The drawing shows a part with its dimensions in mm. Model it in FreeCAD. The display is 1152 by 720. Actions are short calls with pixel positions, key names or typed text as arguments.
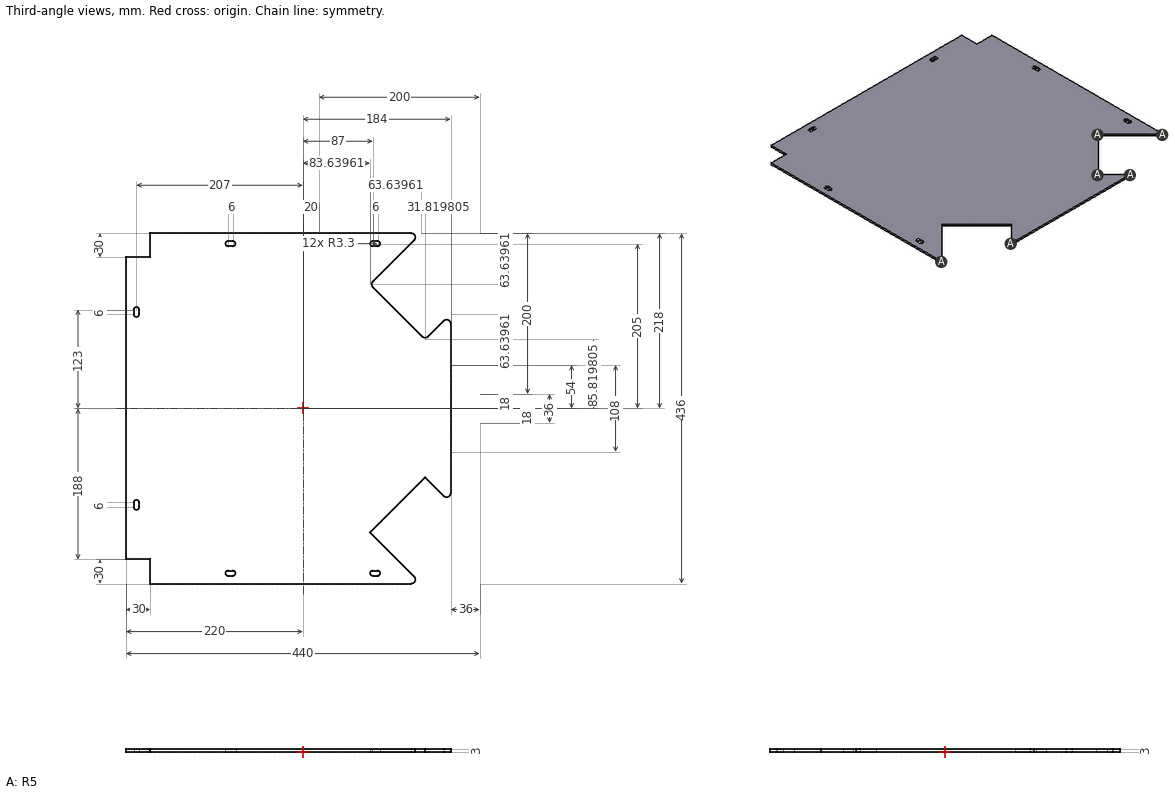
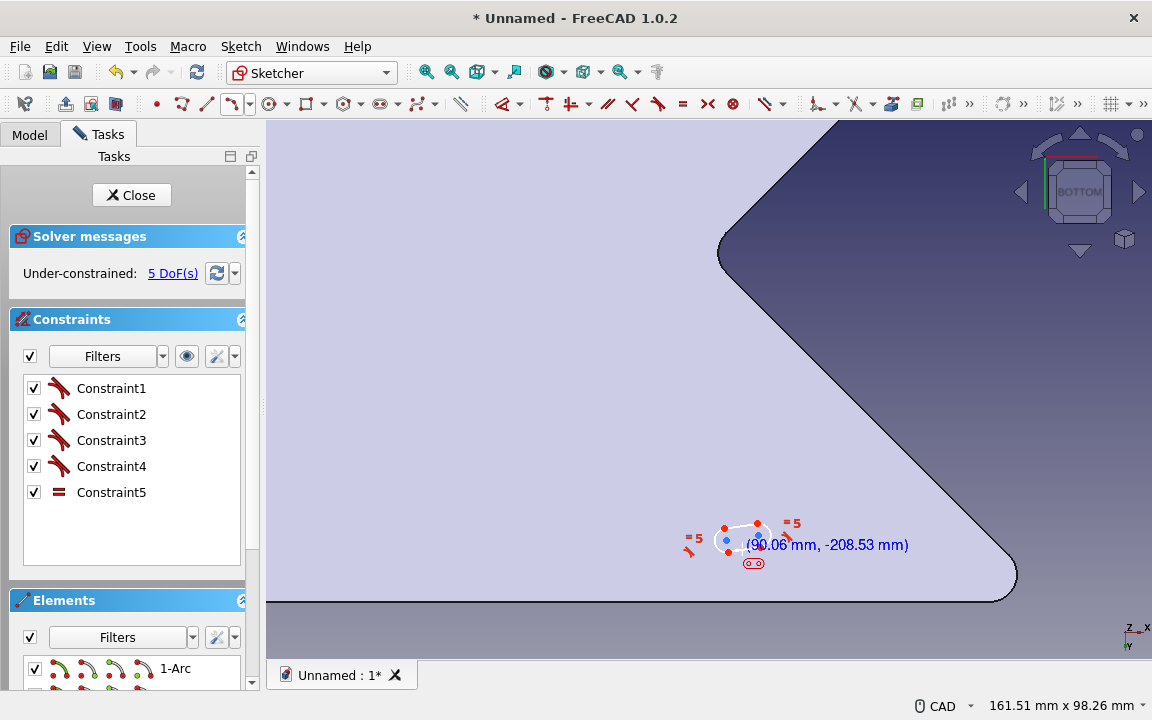
scroll(751, 543, down, 10)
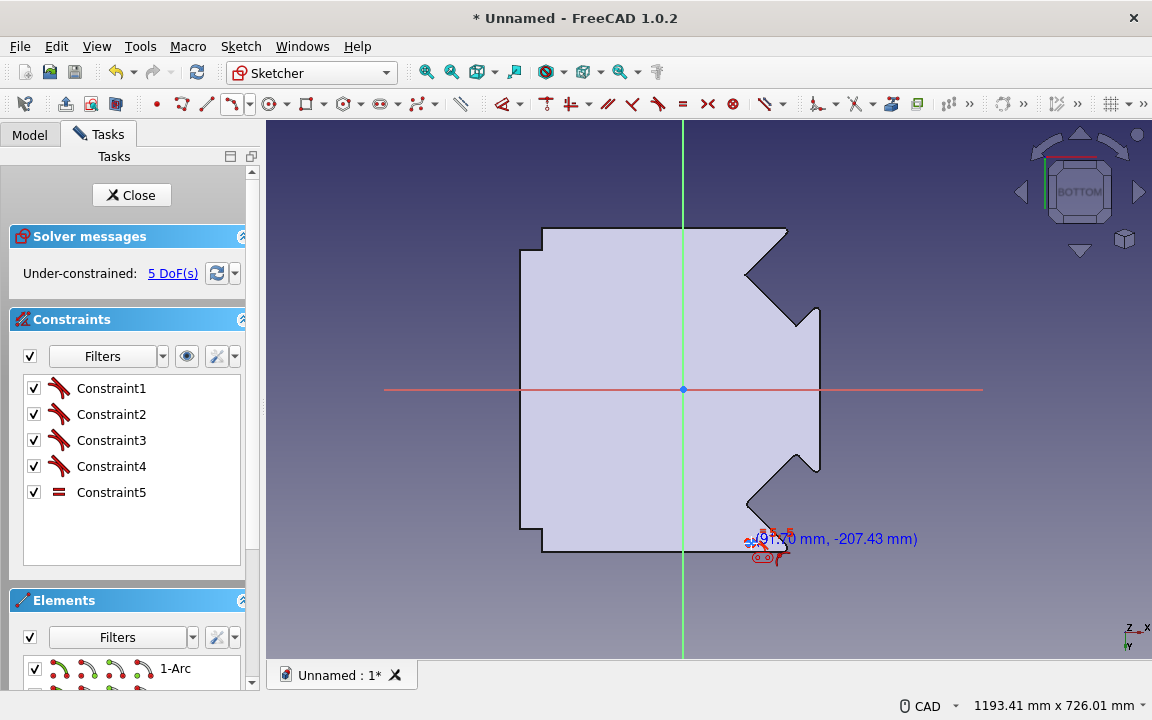
scroll(614, 542, up, 12)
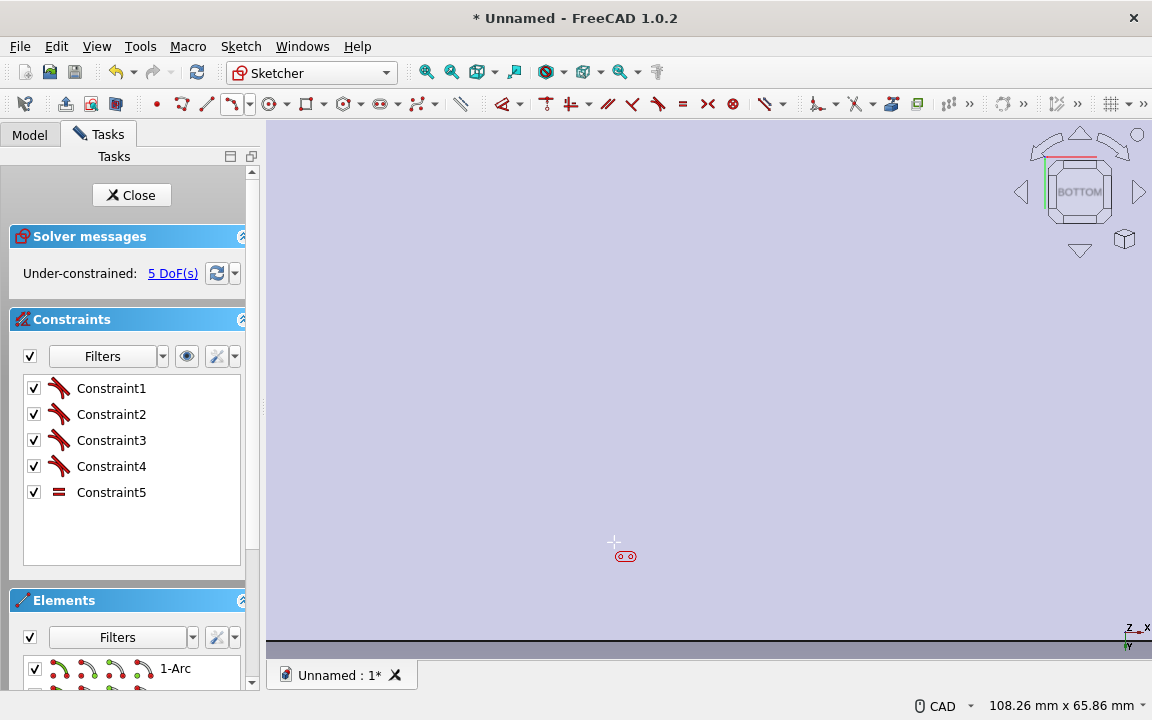
scroll(614, 542, down, 12)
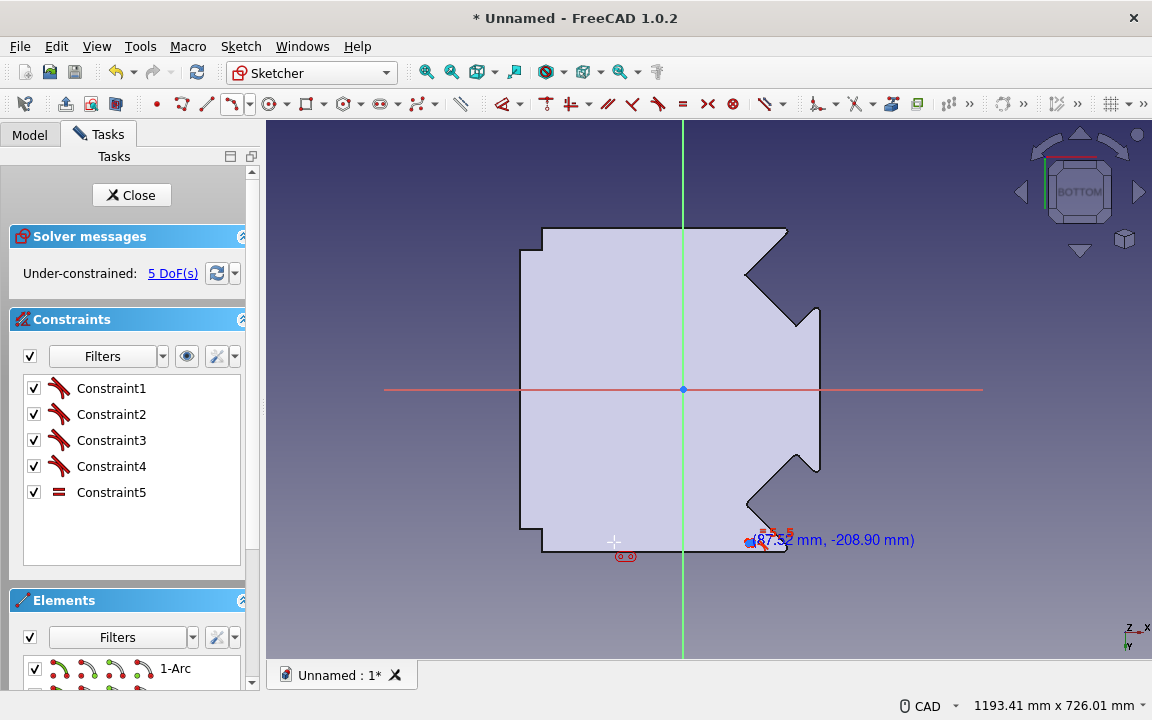
click(614, 542)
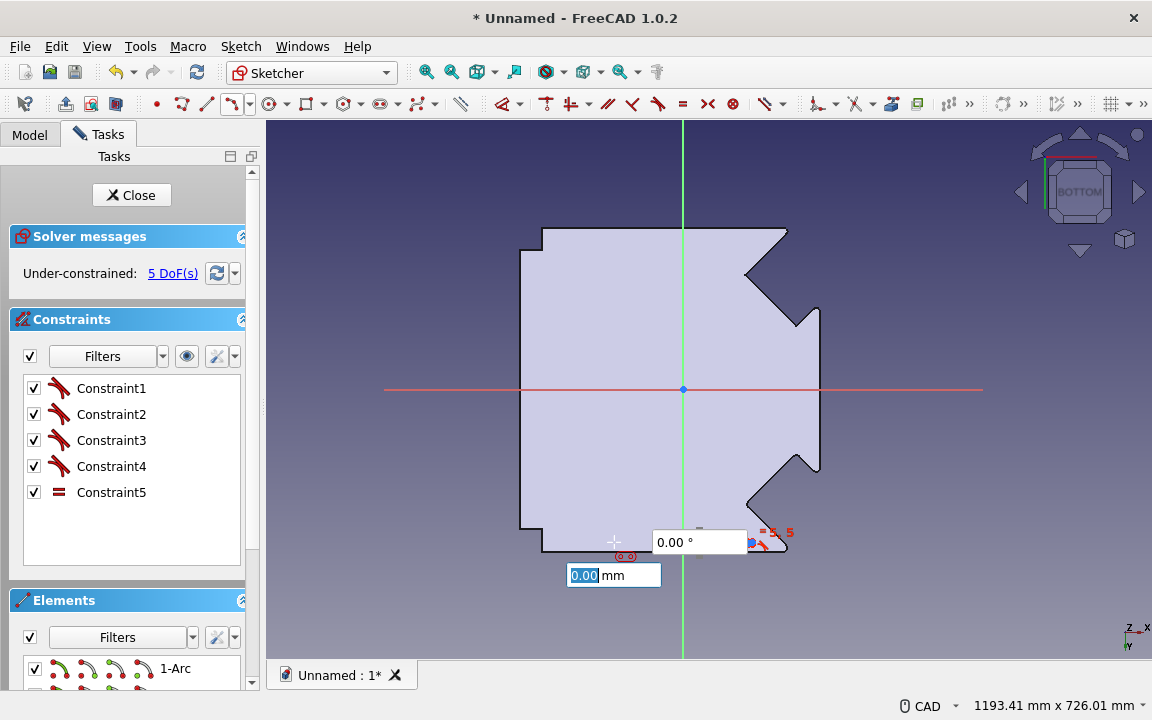
scroll(619, 542, up, 7)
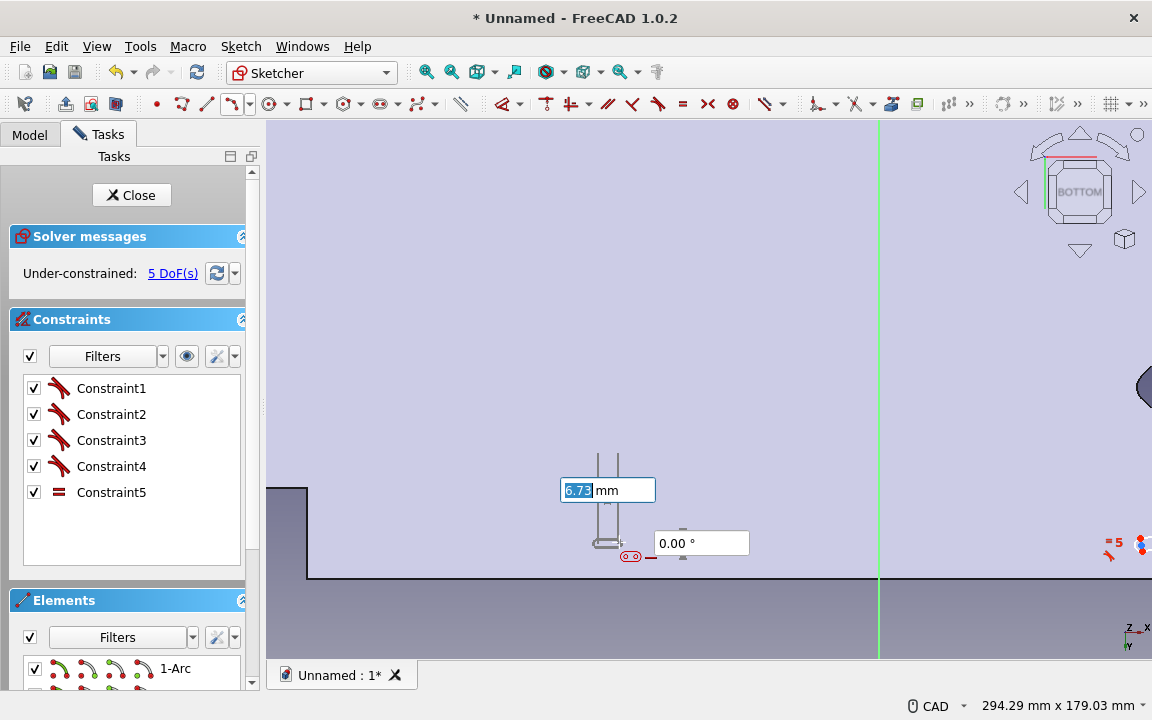
click(617, 540)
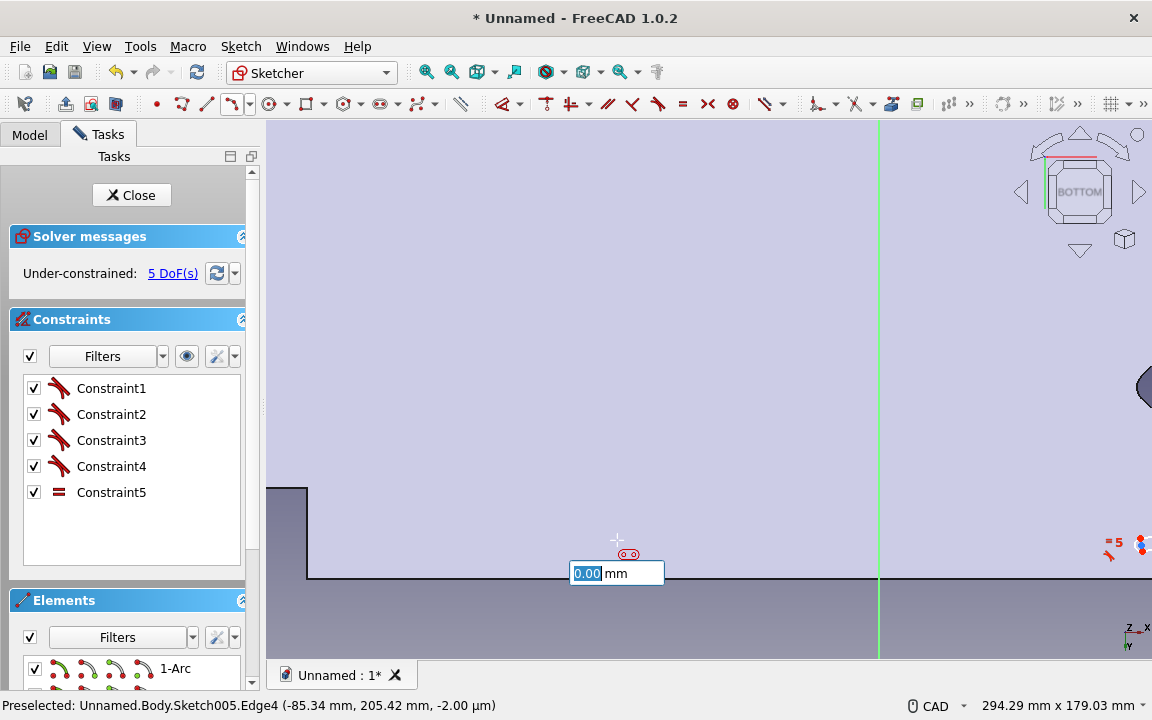
scroll(608, 550, up, 3)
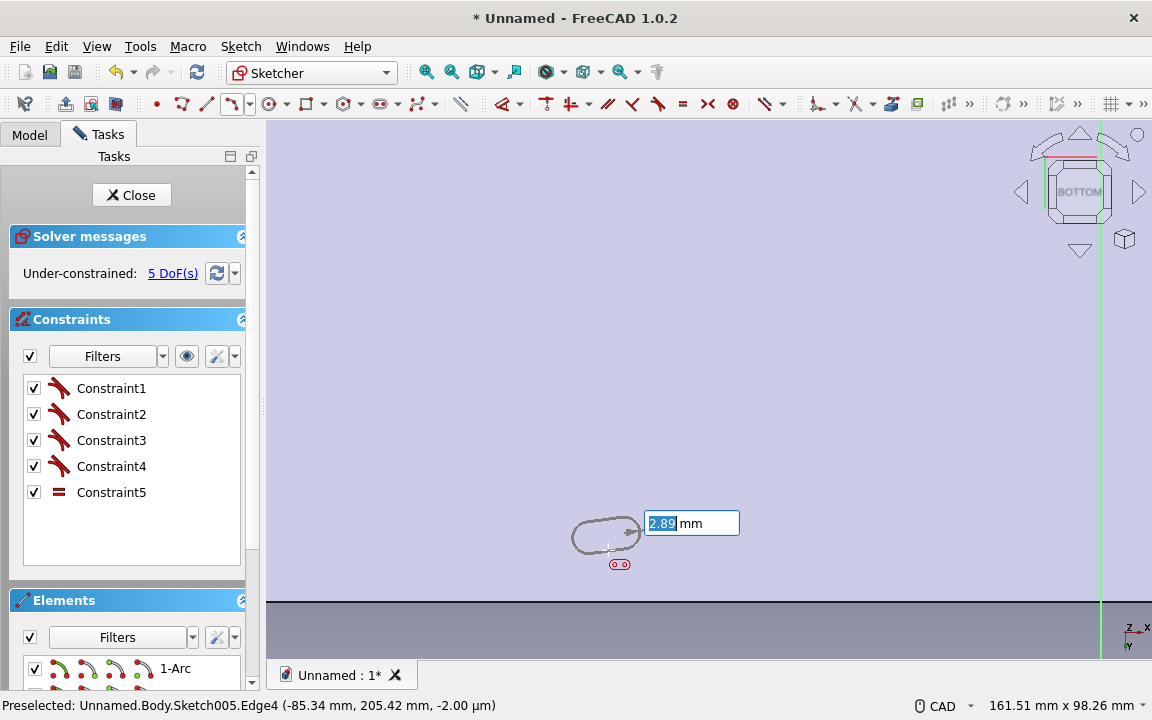
click(608, 549)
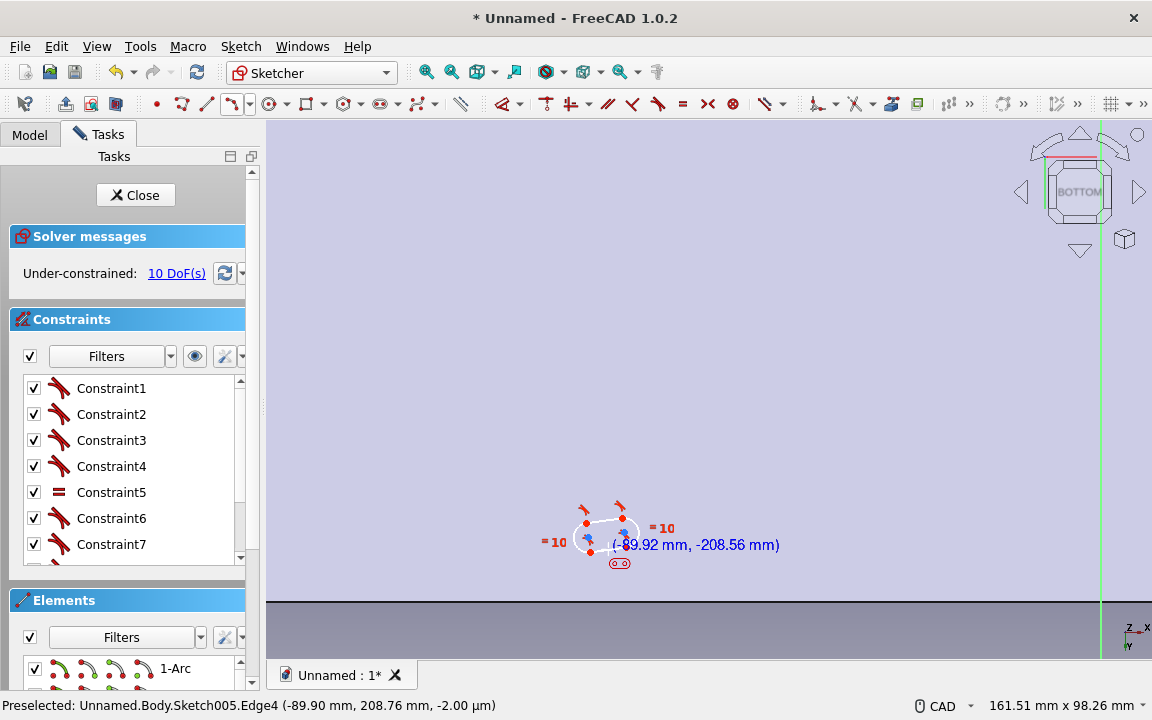
scroll(617, 543, down, 10)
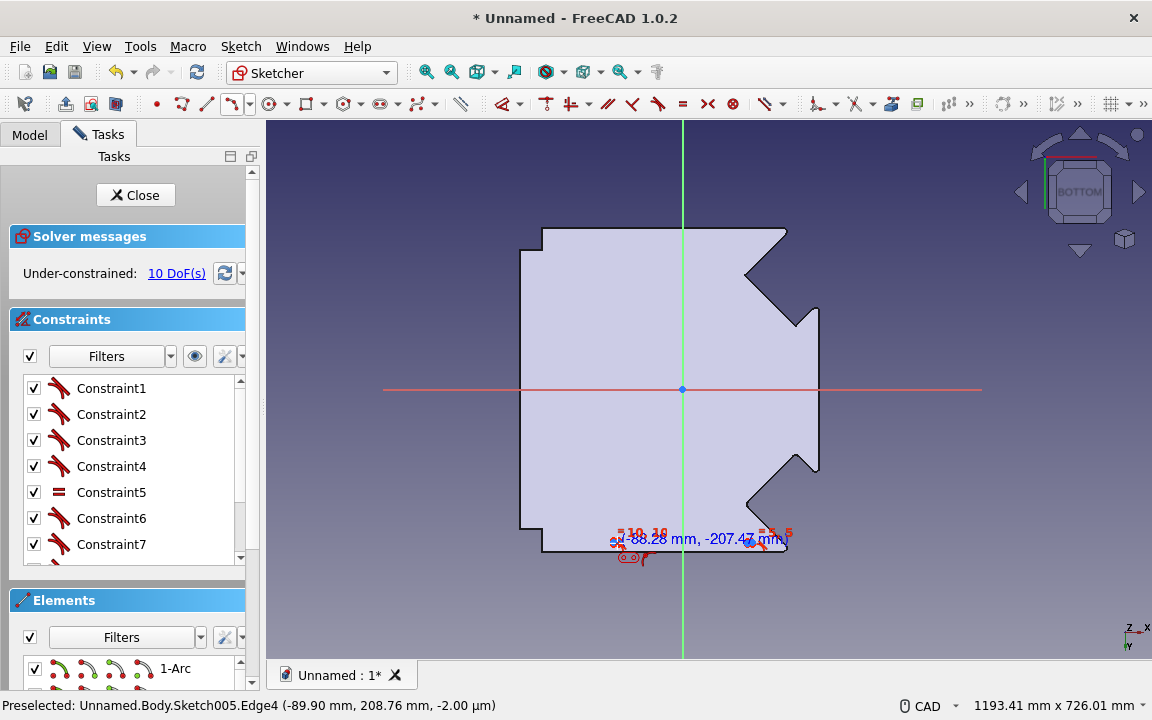
scroll(529, 481, up, 12)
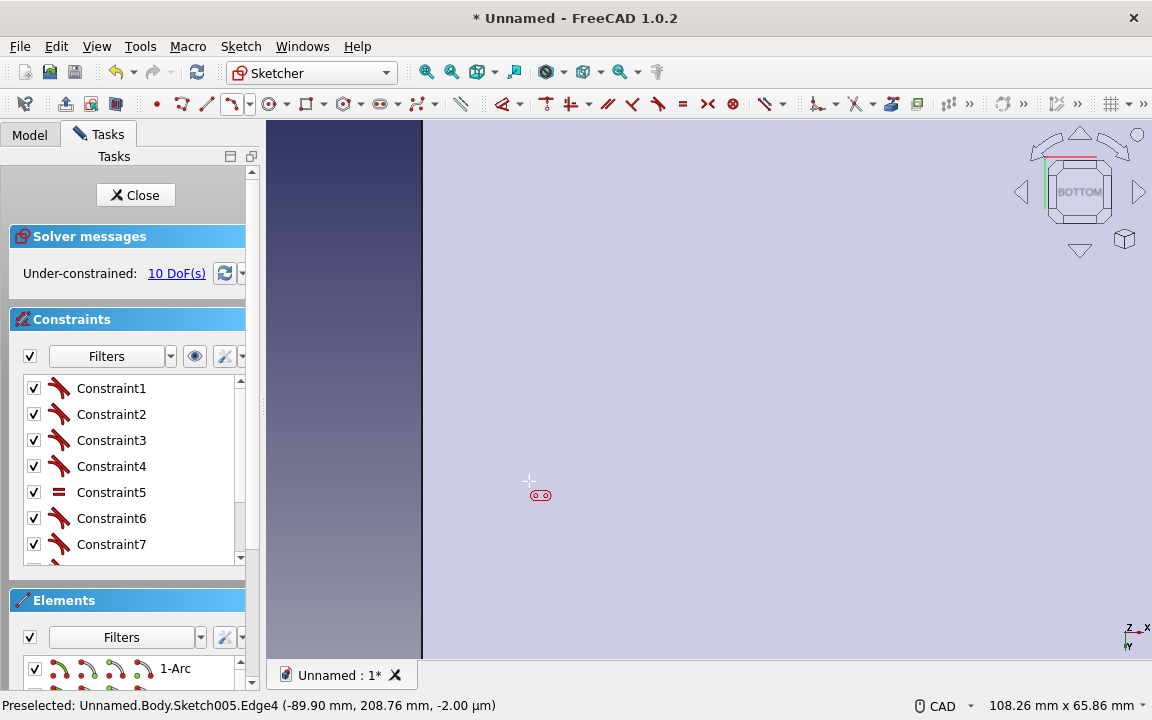
scroll(529, 481, down, 12)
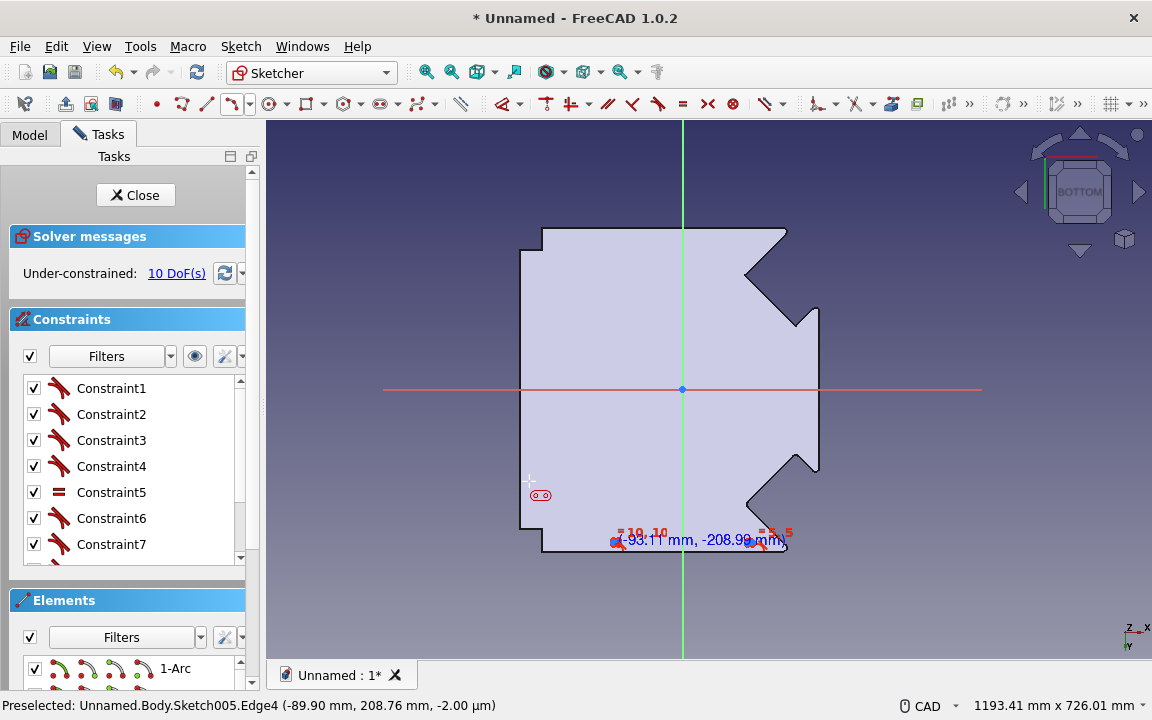
click(529, 481)